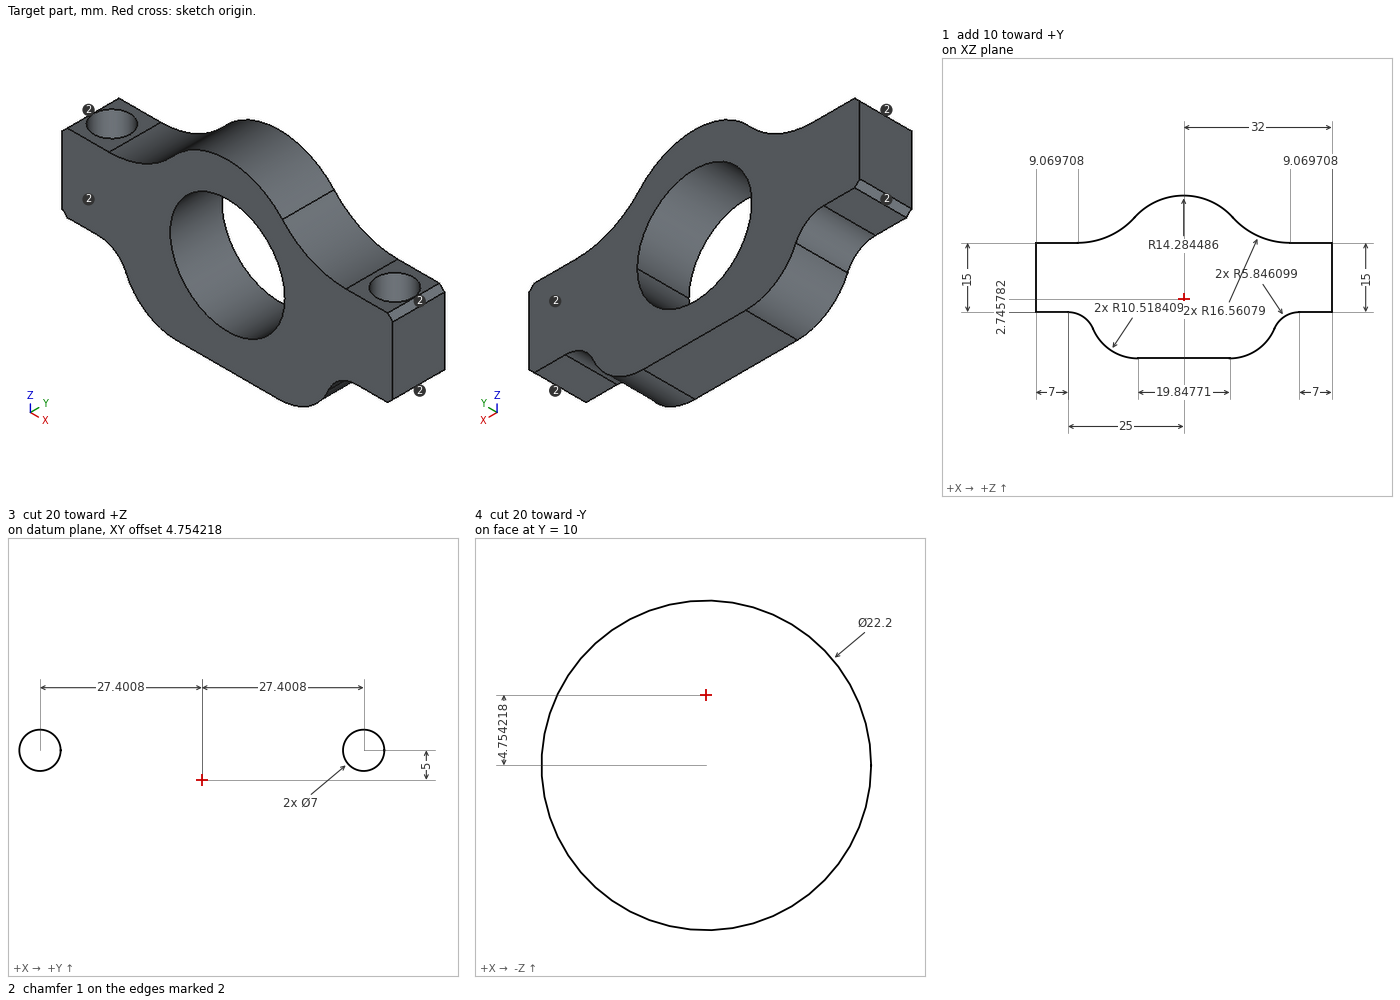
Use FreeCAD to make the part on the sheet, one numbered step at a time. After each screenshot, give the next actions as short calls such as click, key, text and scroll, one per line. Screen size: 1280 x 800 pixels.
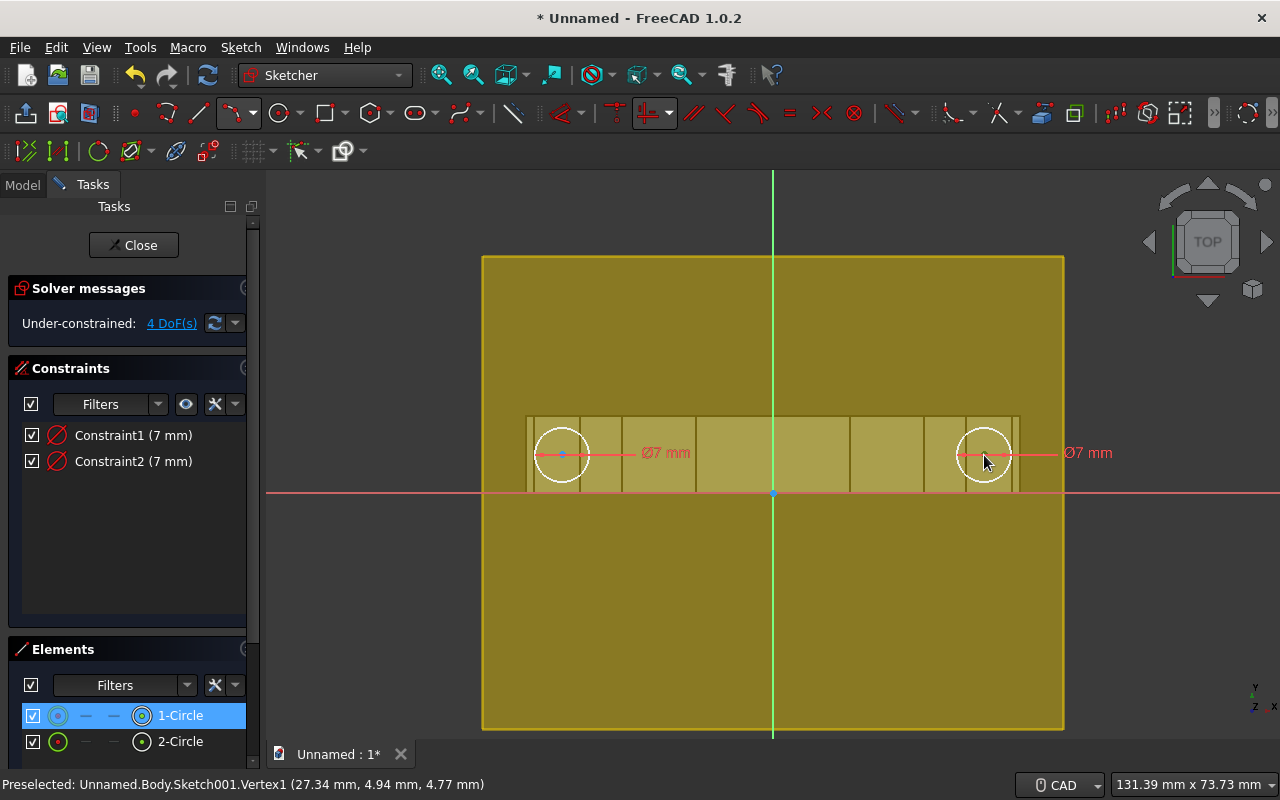
click(562, 455)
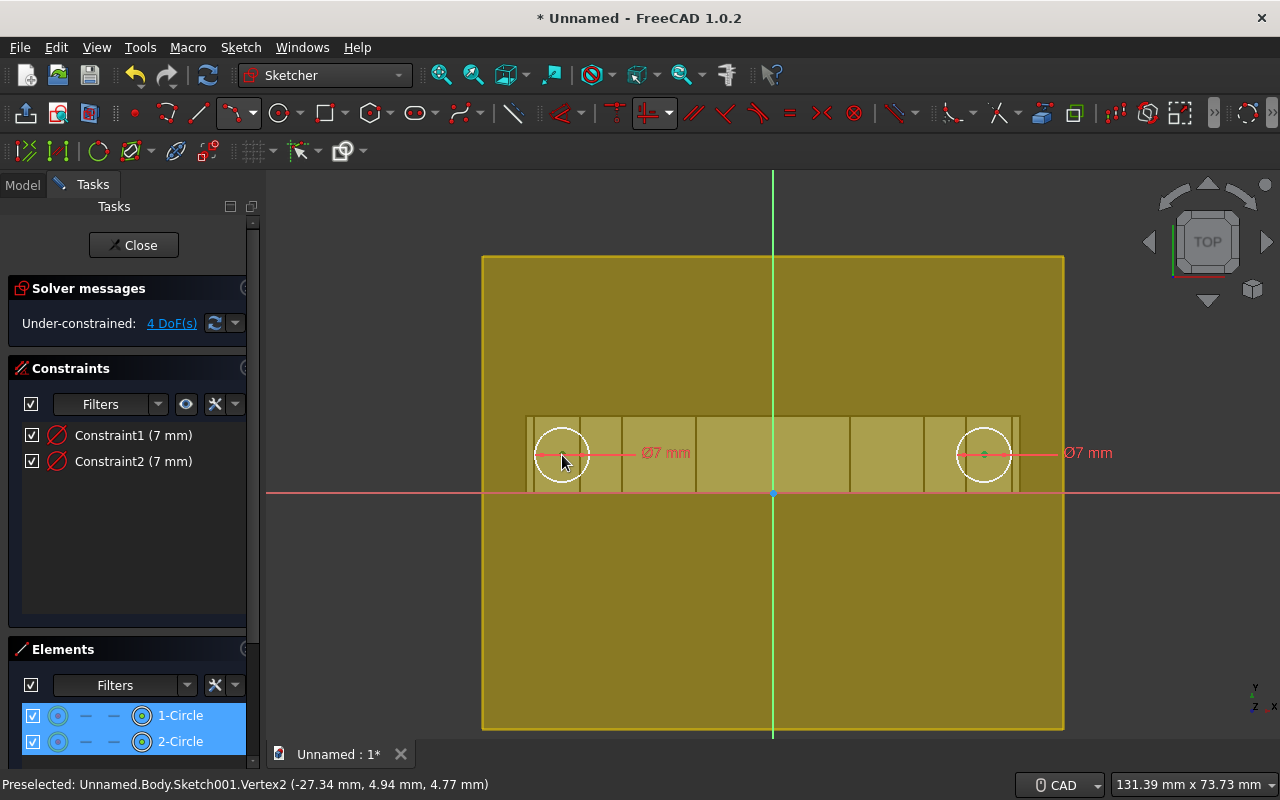
click(672, 114)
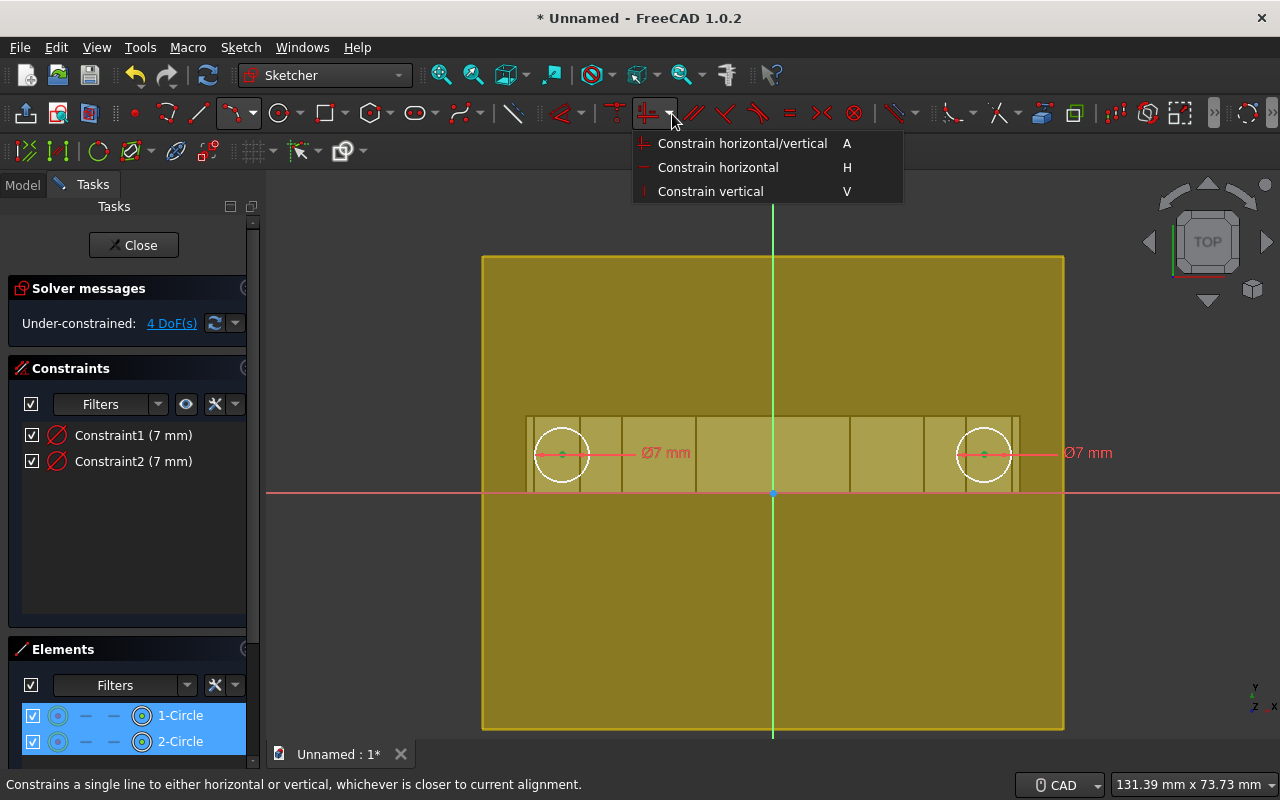
click(768, 167)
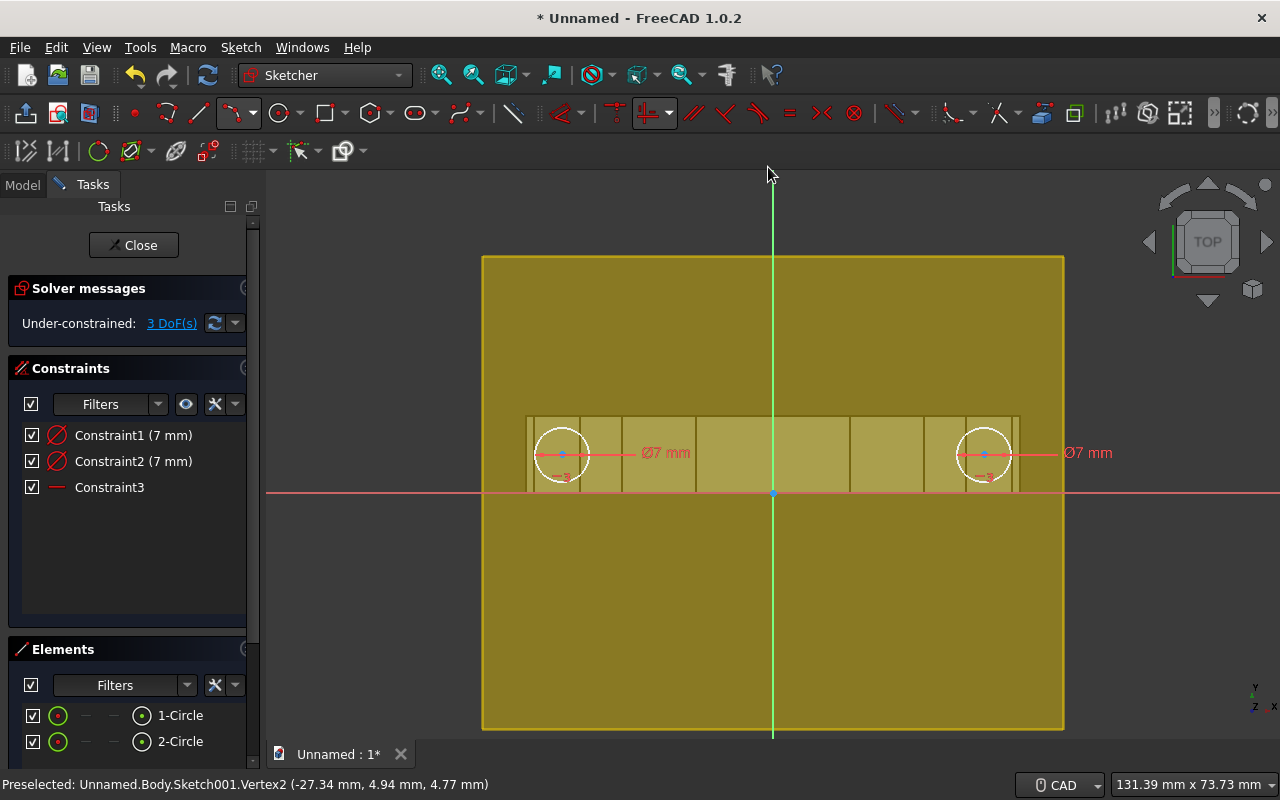
click(560, 114)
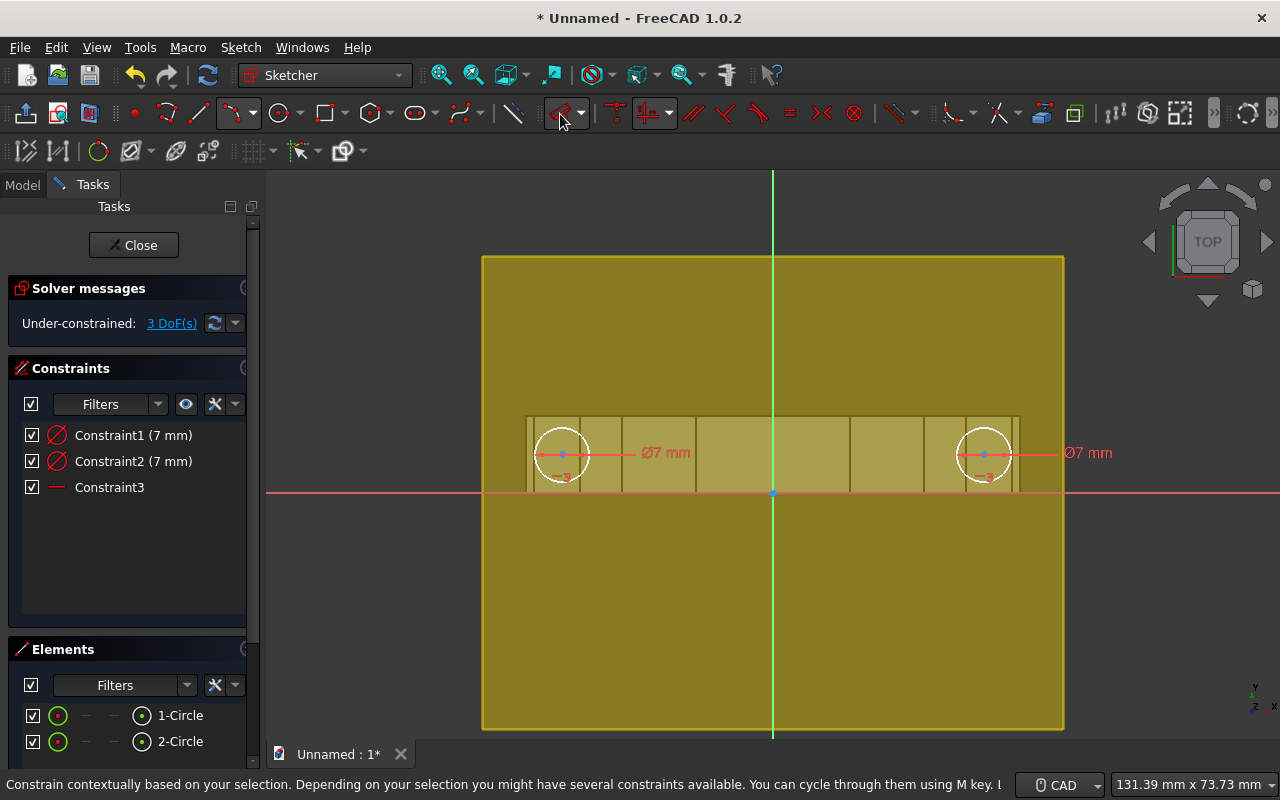
click(984, 455)
click(739, 474)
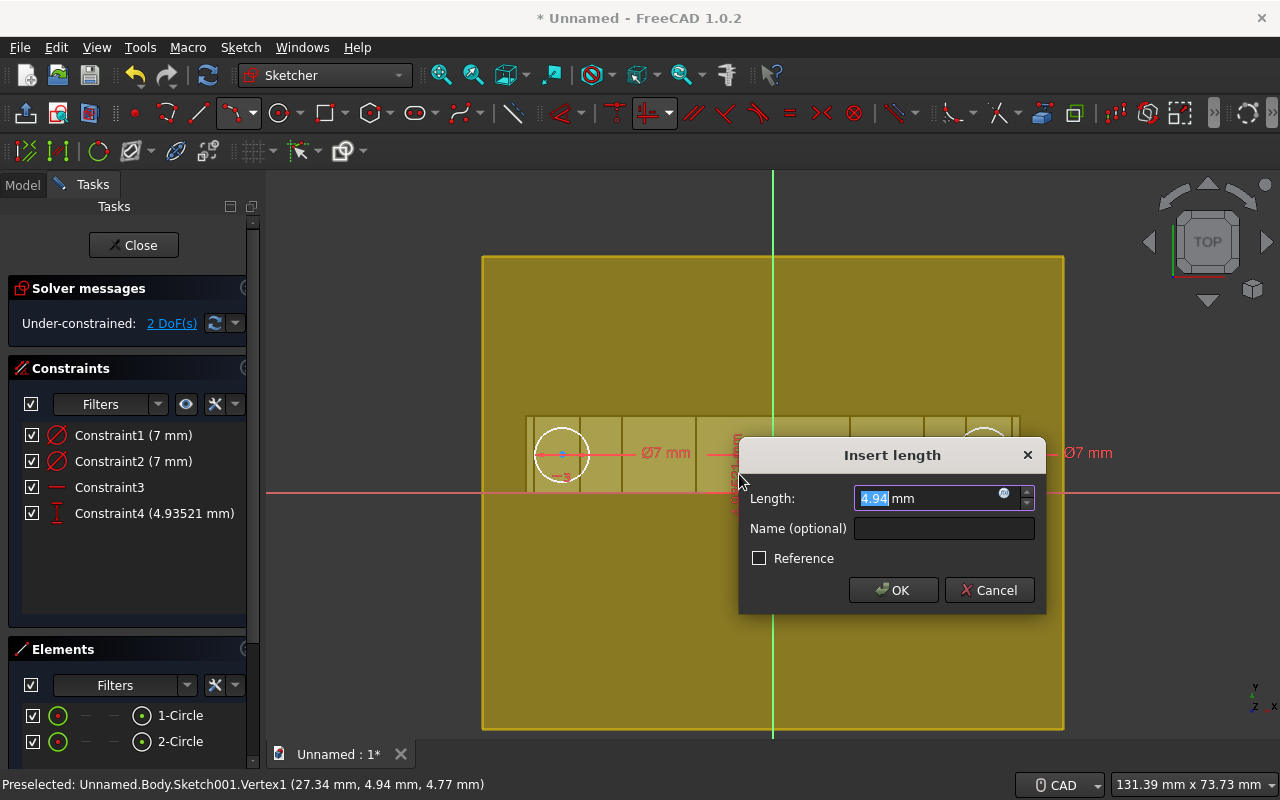
text(5)
key(Return)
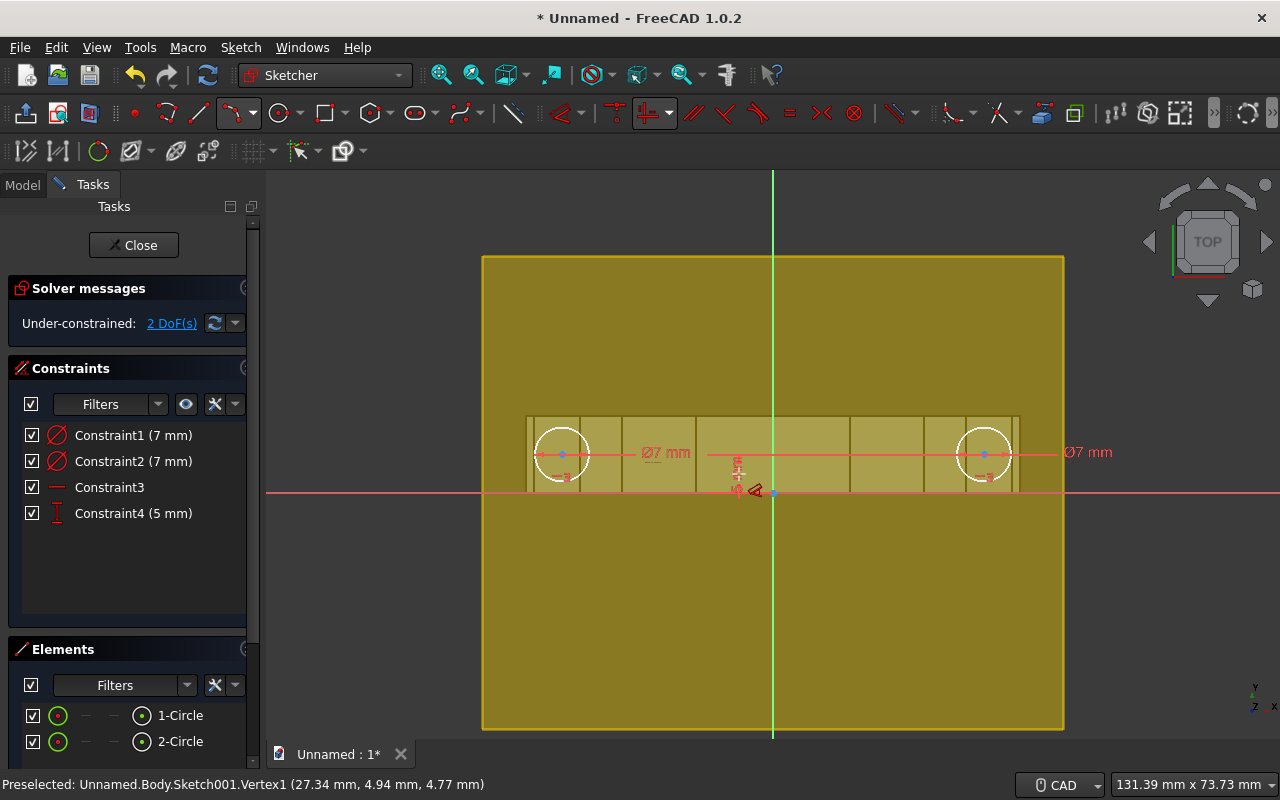
click(984, 454)
click(878, 527)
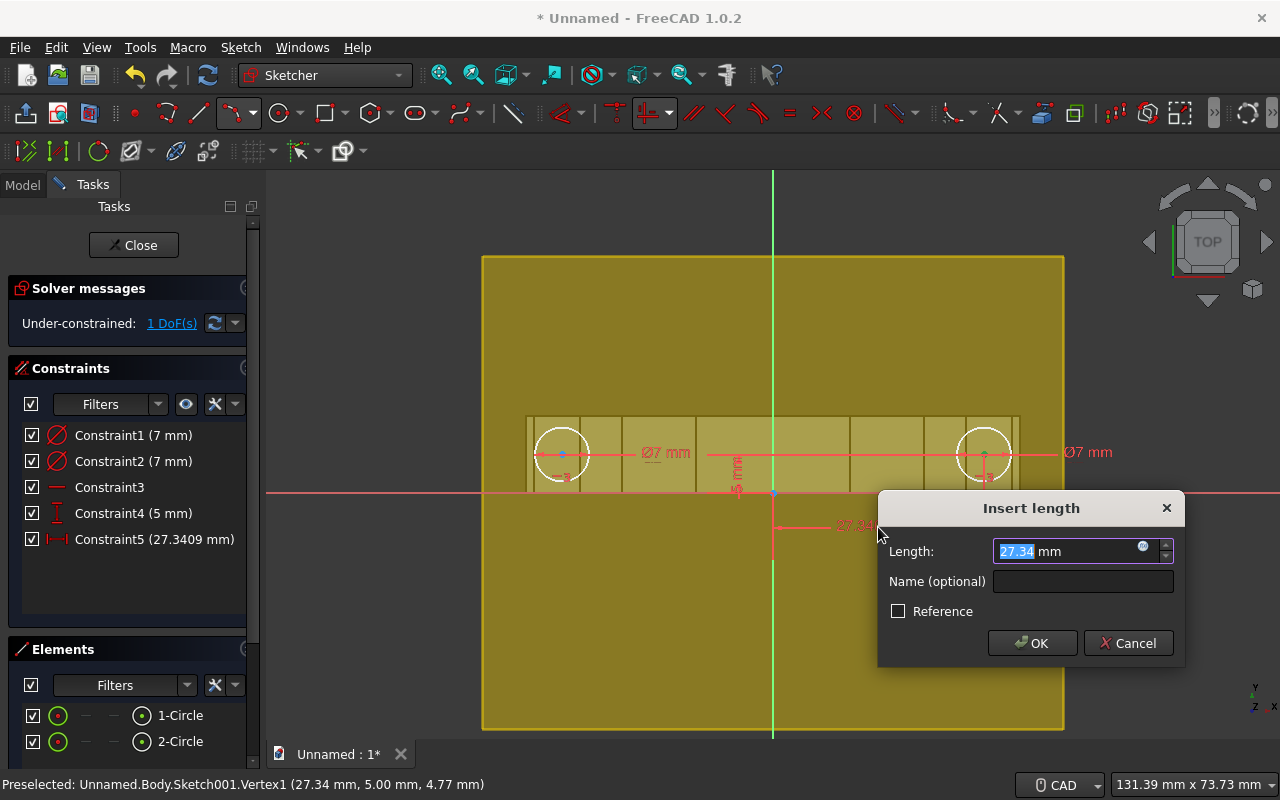
text(27.4008)
key(Return)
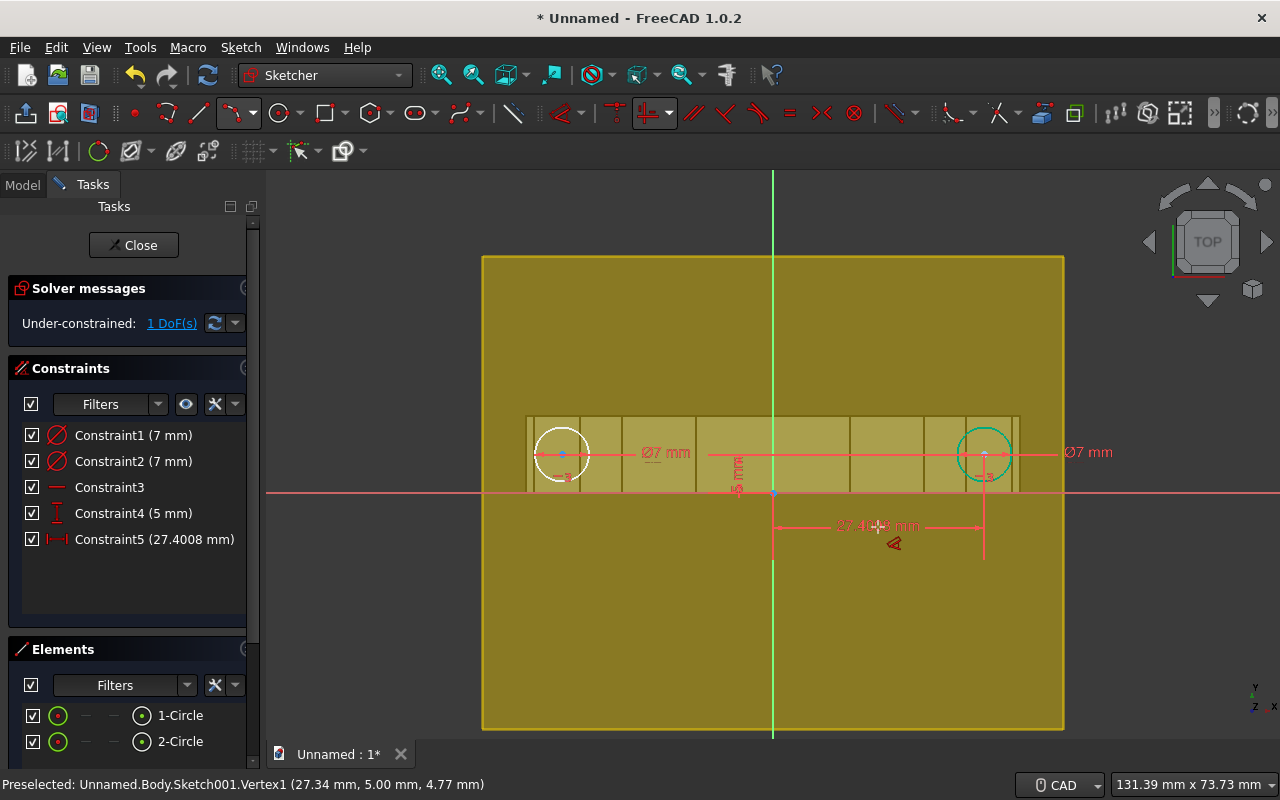
click(562, 454)
click(667, 527)